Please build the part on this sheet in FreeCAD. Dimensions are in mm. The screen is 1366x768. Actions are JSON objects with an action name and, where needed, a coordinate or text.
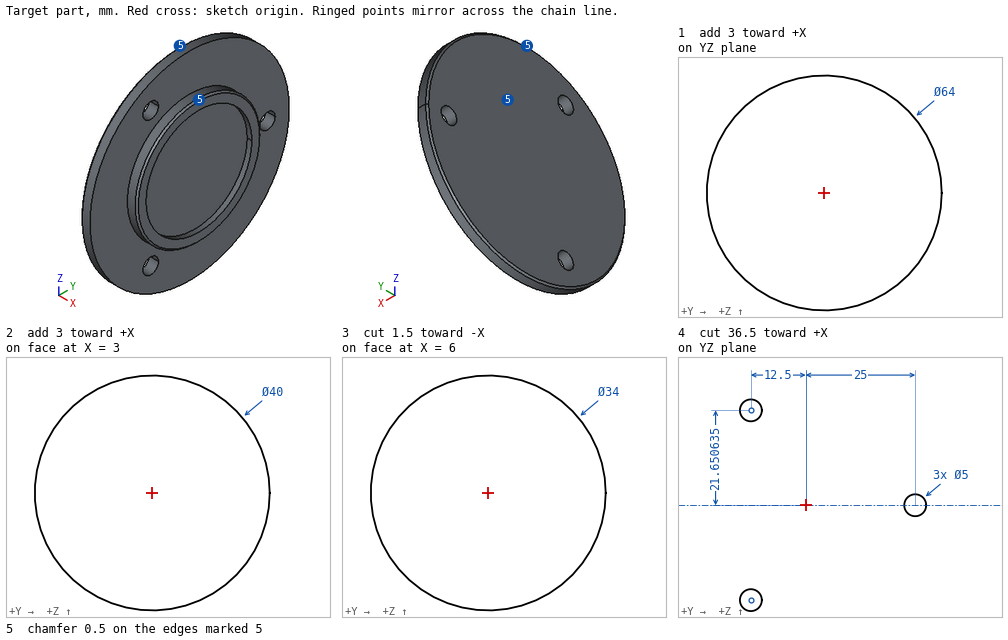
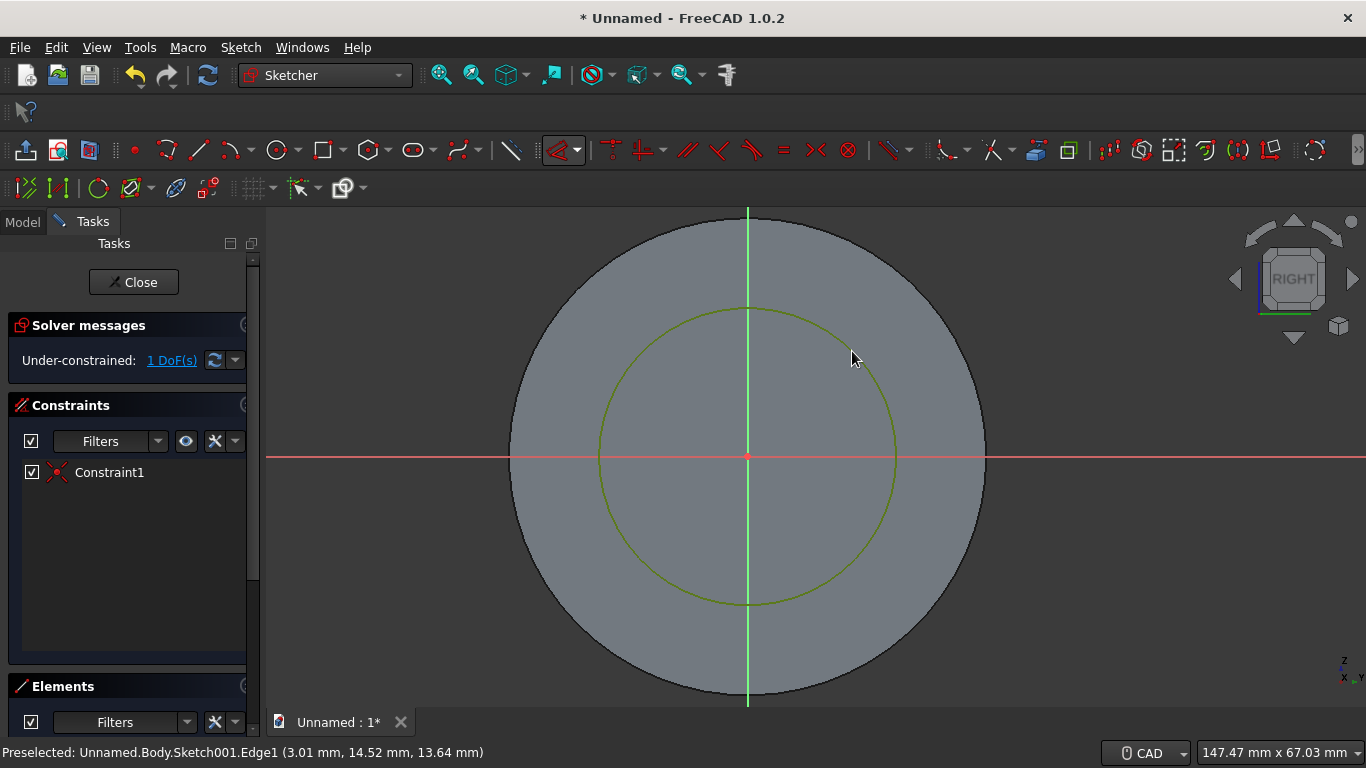
{"action": "left_click", "coordinate": [580, 150]}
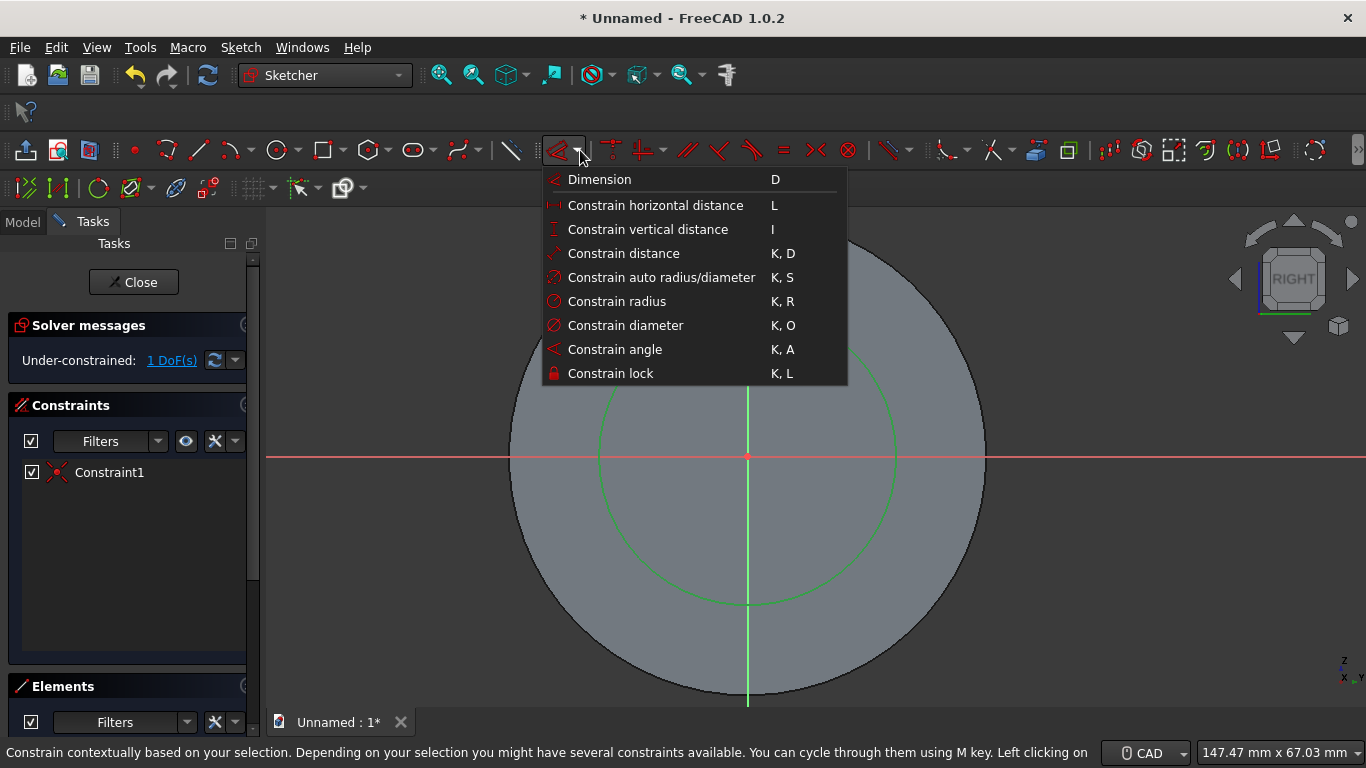
{"action": "left_click", "coordinate": [695, 325]}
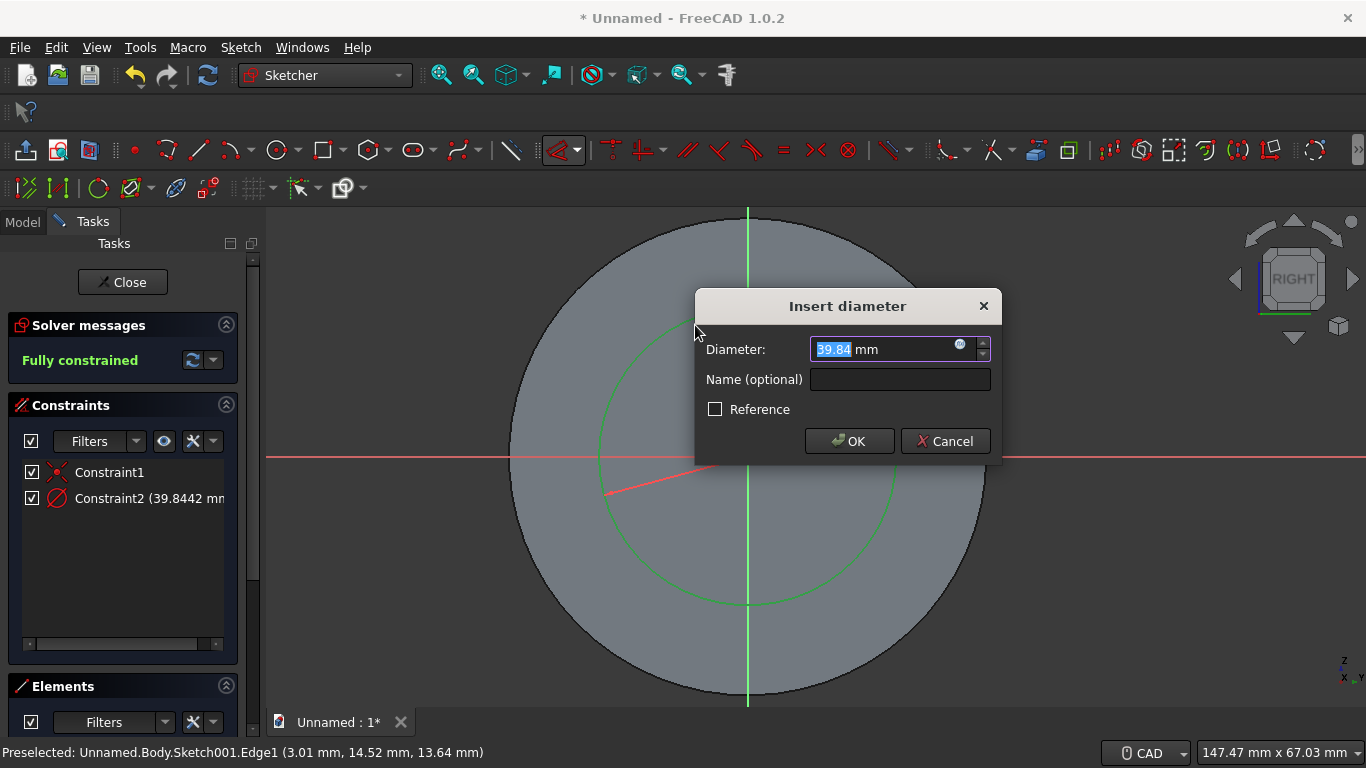
{"action": "type", "text": "40"}
{"action": "key", "text": "Return"}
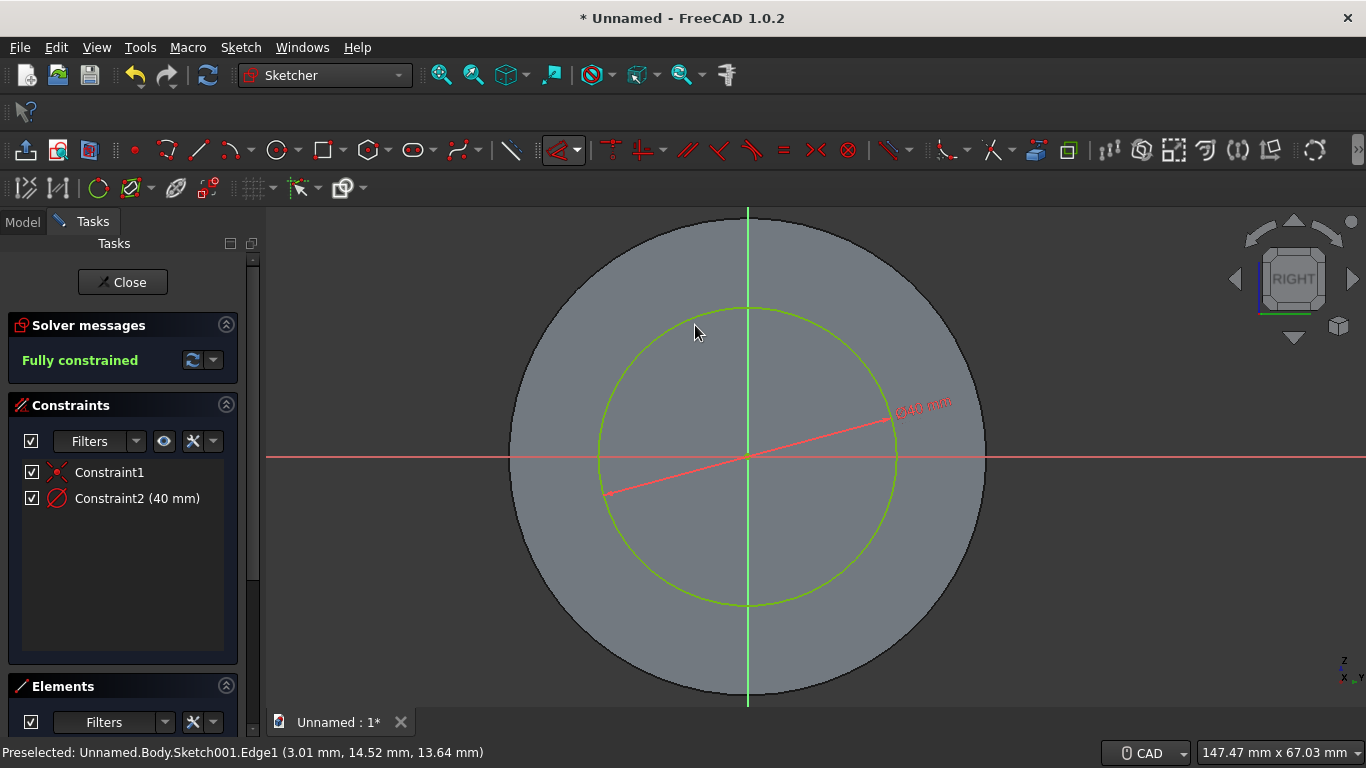
{"action": "left_click", "coordinate": [123, 282]}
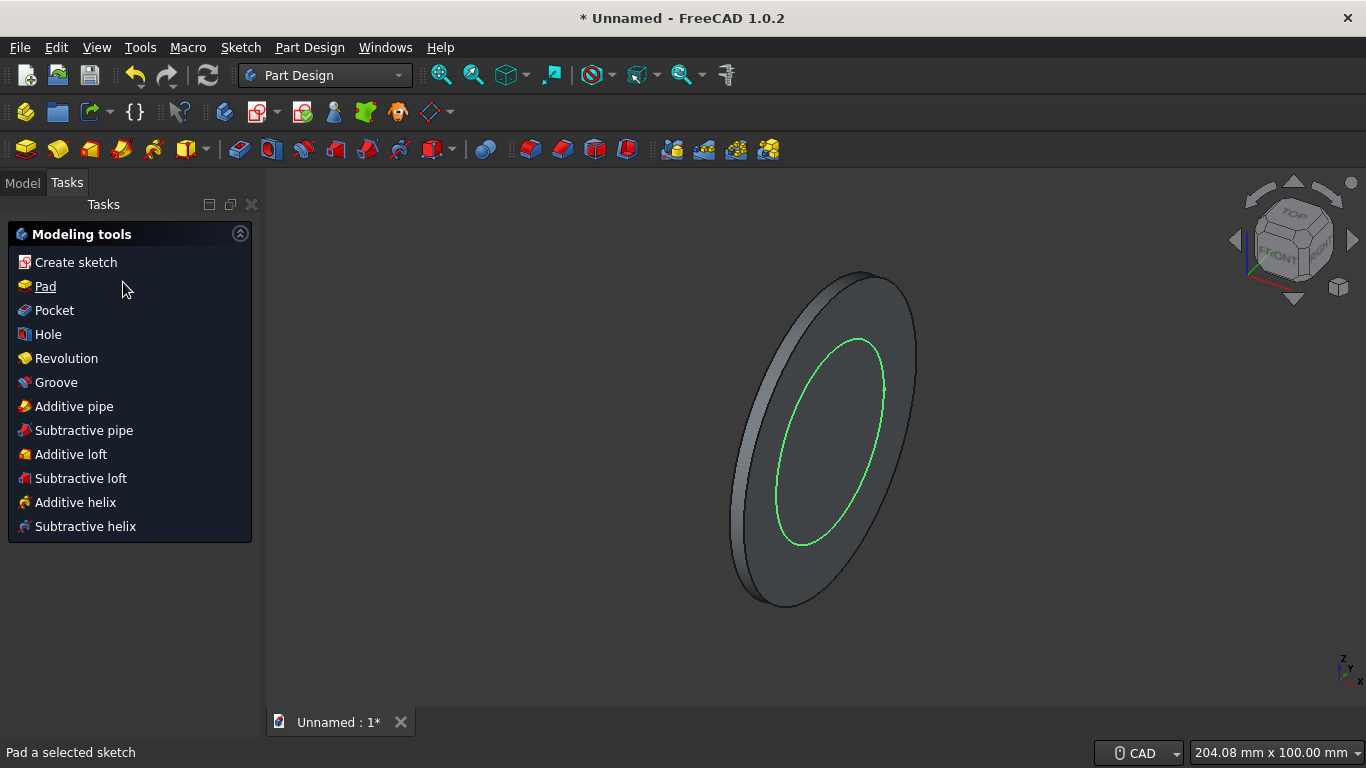
{"action": "left_click", "coordinate": [26, 150]}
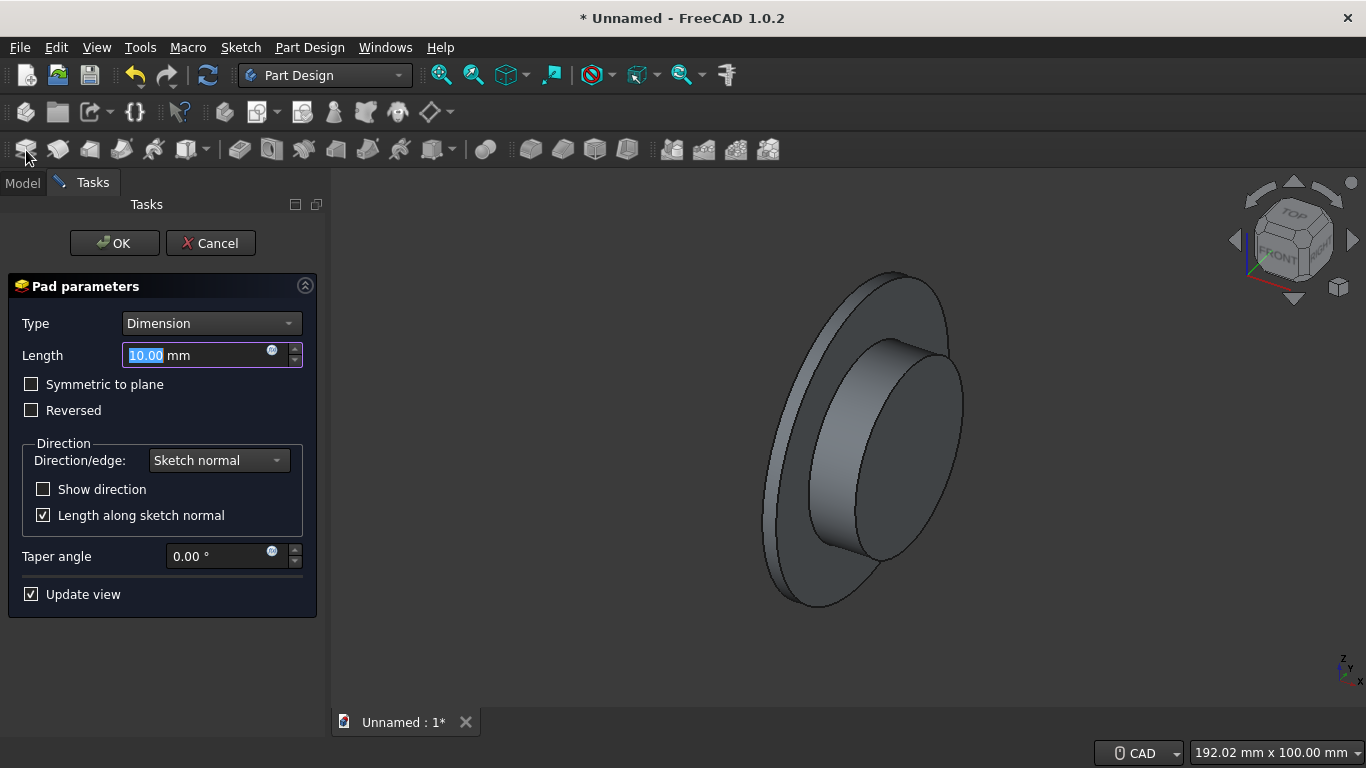
{"action": "type", "text": "3"}
{"action": "key", "text": "Tab"}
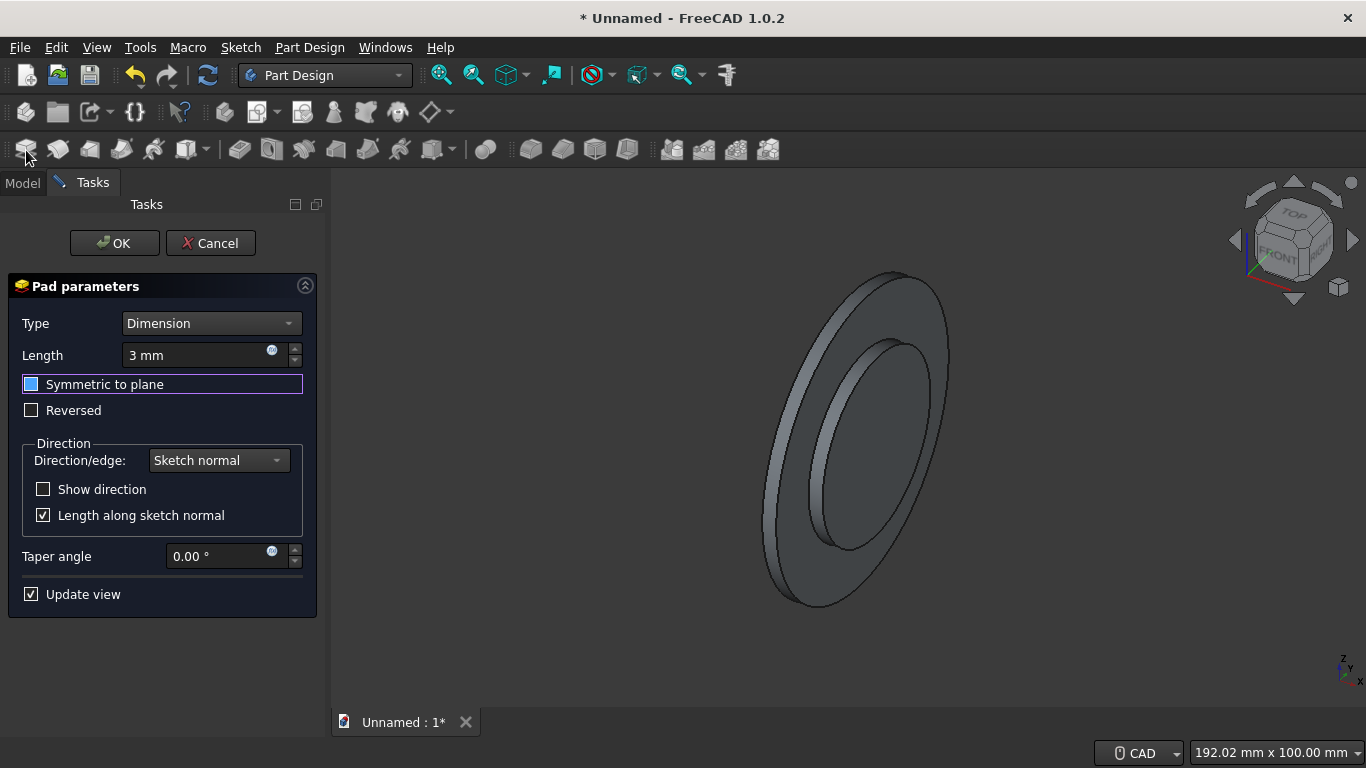
{"action": "left_click", "coordinate": [115, 243]}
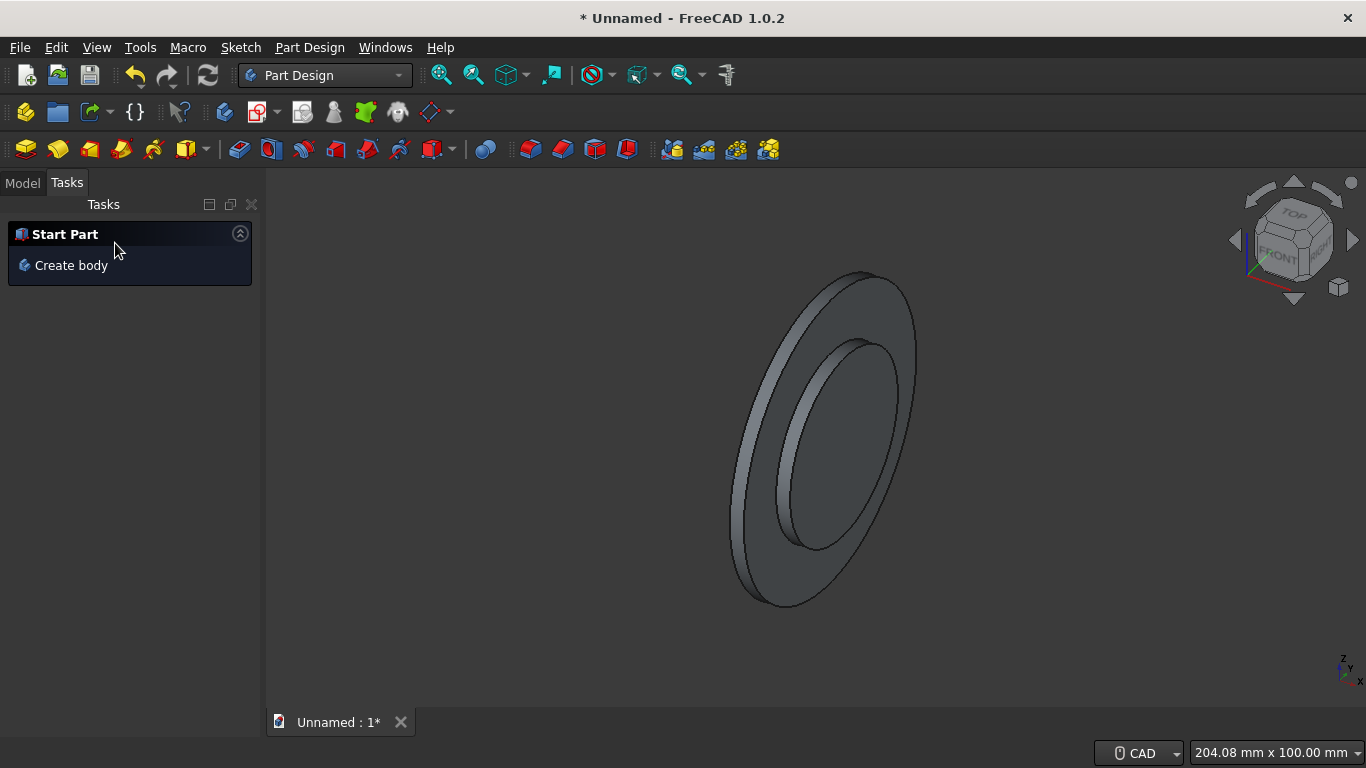
{"action": "left_click", "coordinate": [844, 446]}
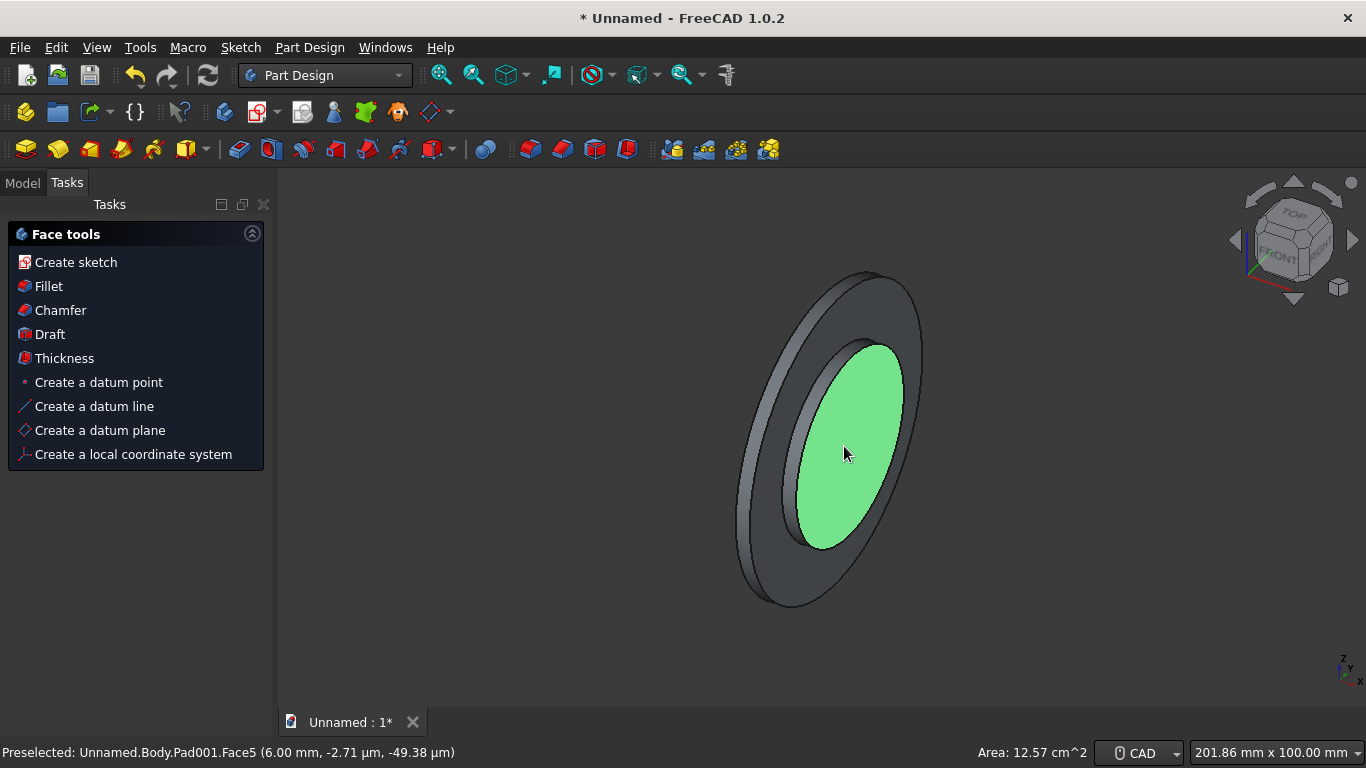
{"action": "left_click", "coordinate": [258, 112]}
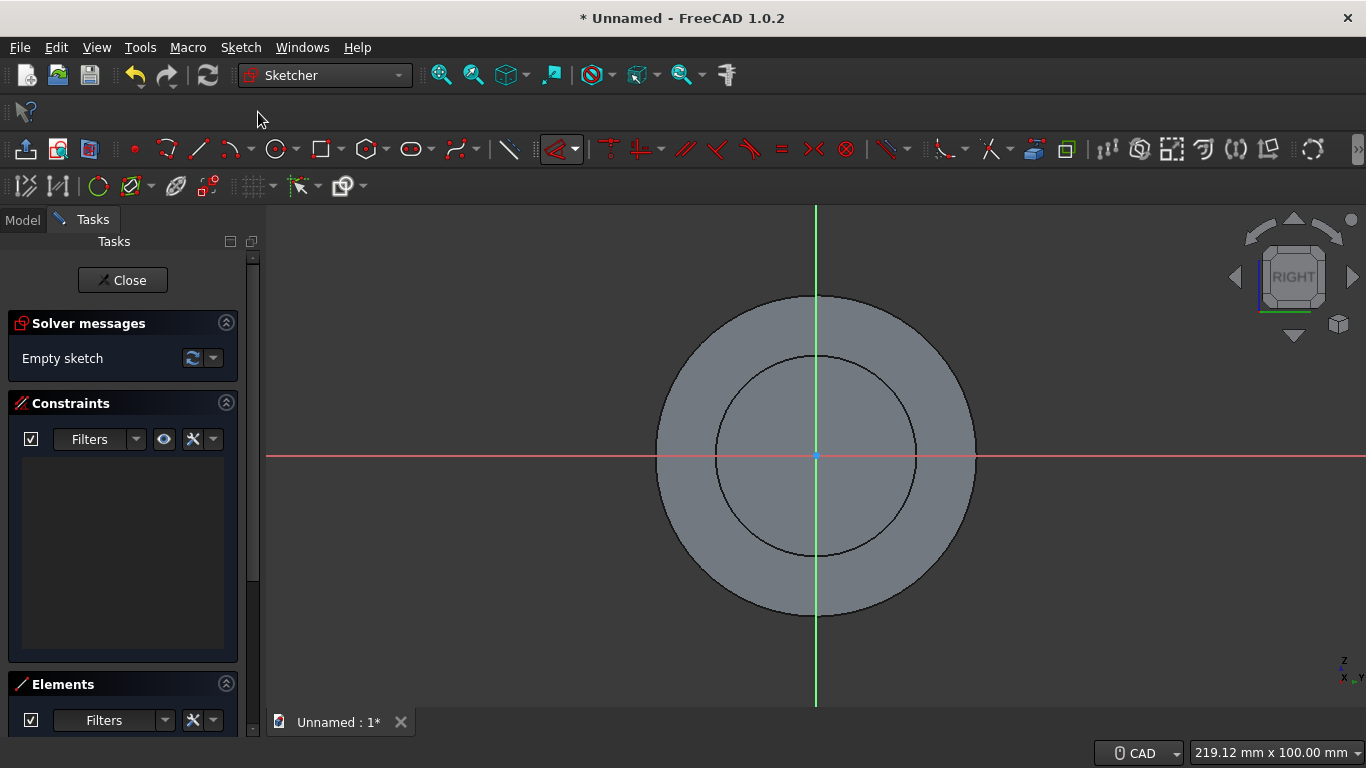
{"action": "scroll", "coordinate": [899, 456], "scroll_direction": "up", "scroll_amount": 3}